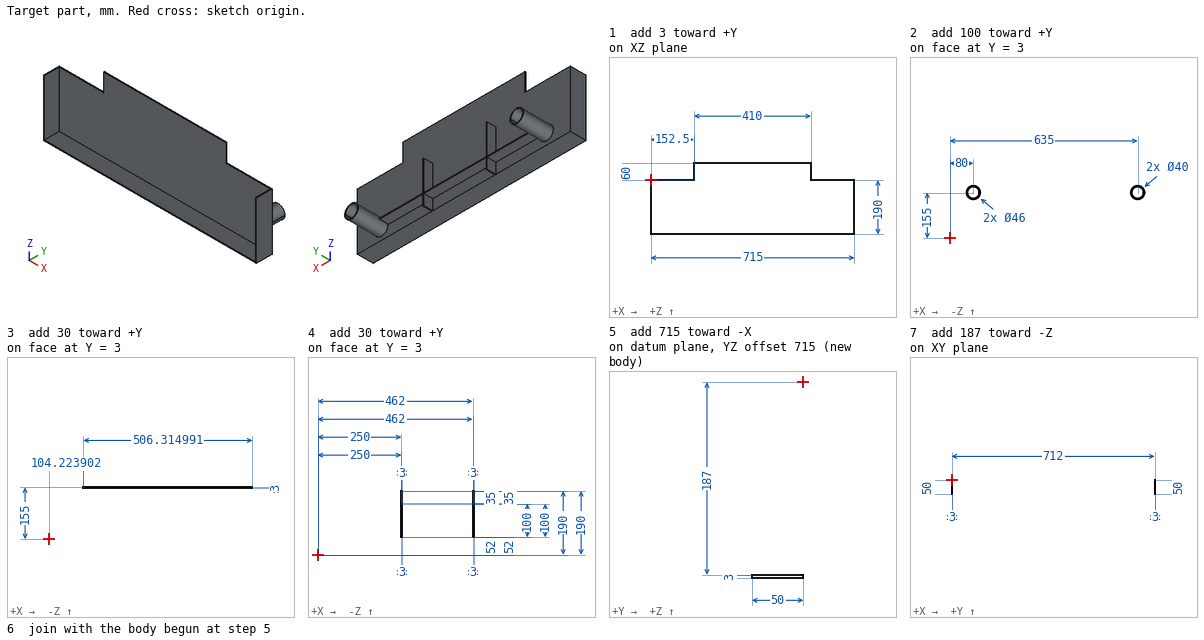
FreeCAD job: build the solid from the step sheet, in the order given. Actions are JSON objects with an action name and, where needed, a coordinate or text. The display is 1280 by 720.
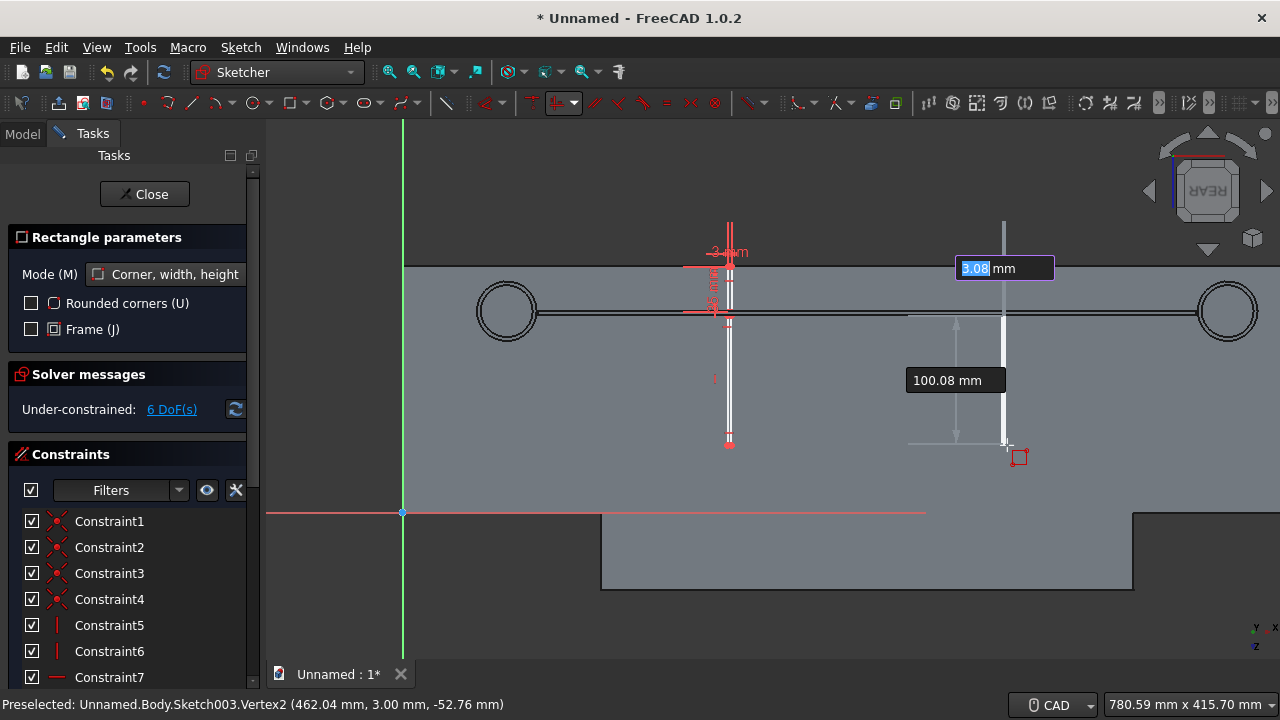
{"action": "type", "text": "3"}
{"action": "key", "text": "Tab"}
{"action": "type", "text": "100"}
{"action": "key", "text": "Return"}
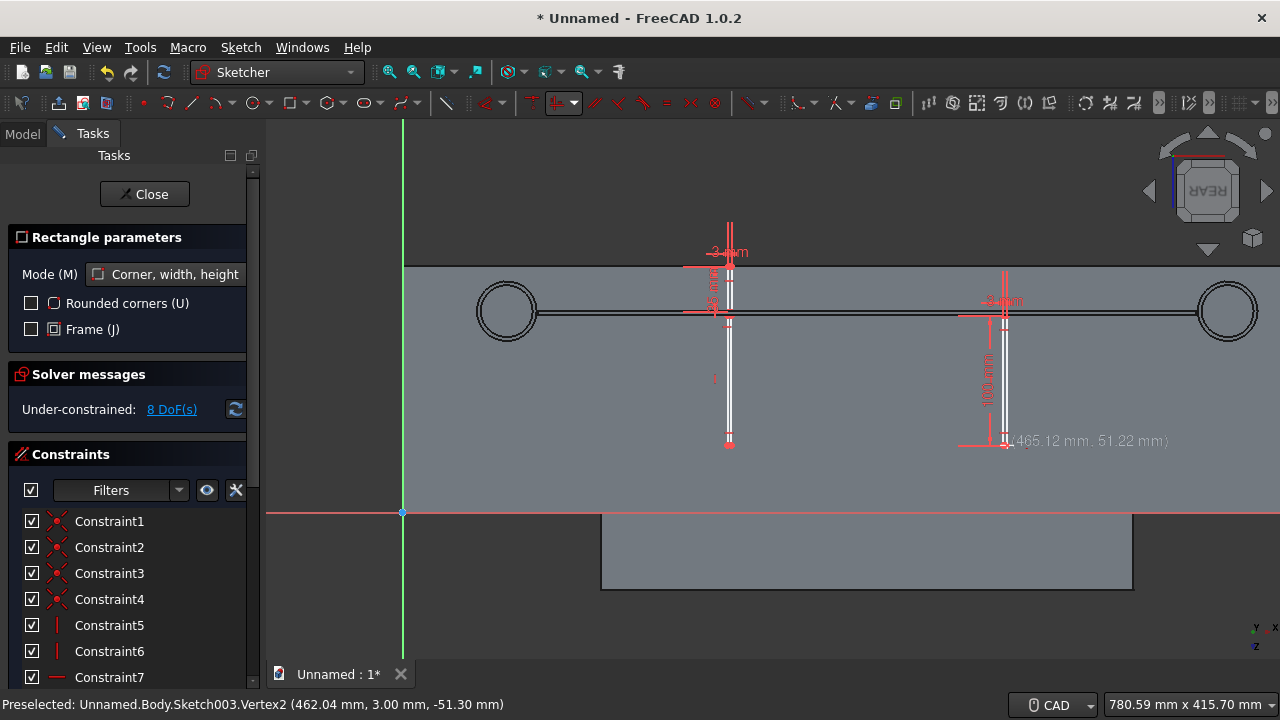
{"action": "scroll", "coordinate": [1003, 266], "scroll_direction": "up", "scroll_amount": 8}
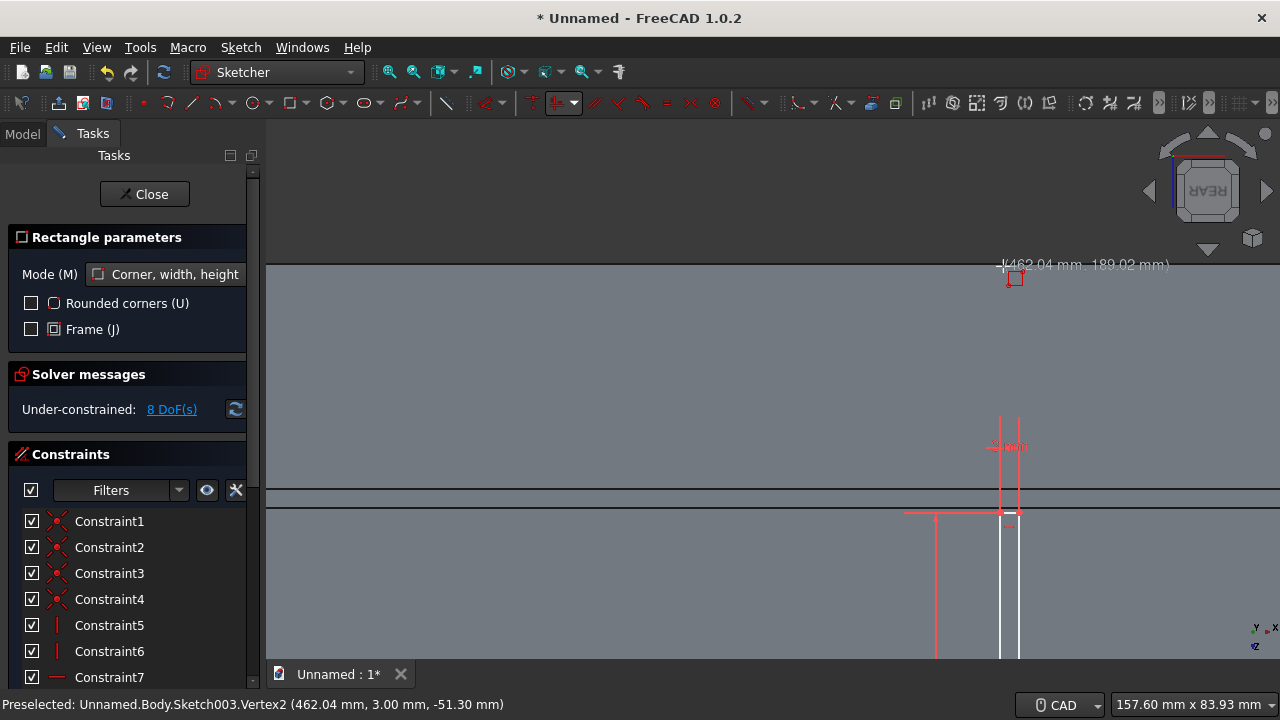
{"action": "scroll", "coordinate": [1003, 266], "scroll_direction": "down", "scroll_amount": 8}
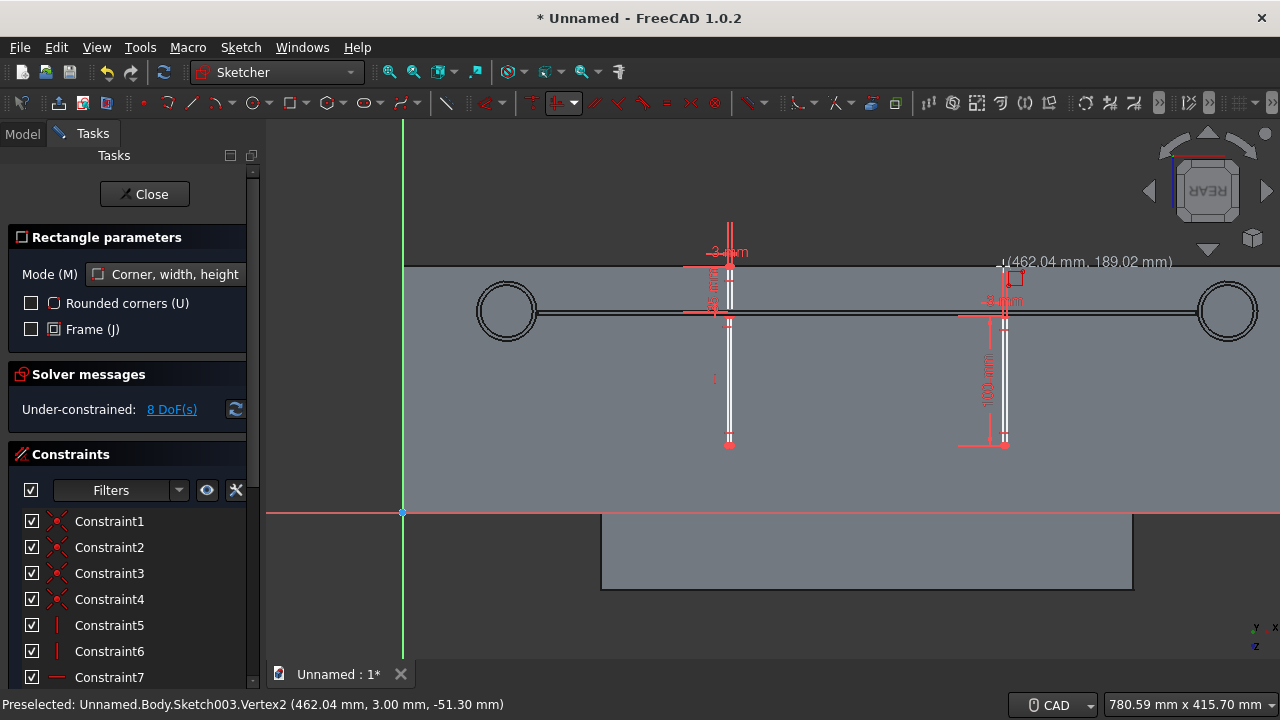
{"action": "left_click", "coordinate": [1003, 266]}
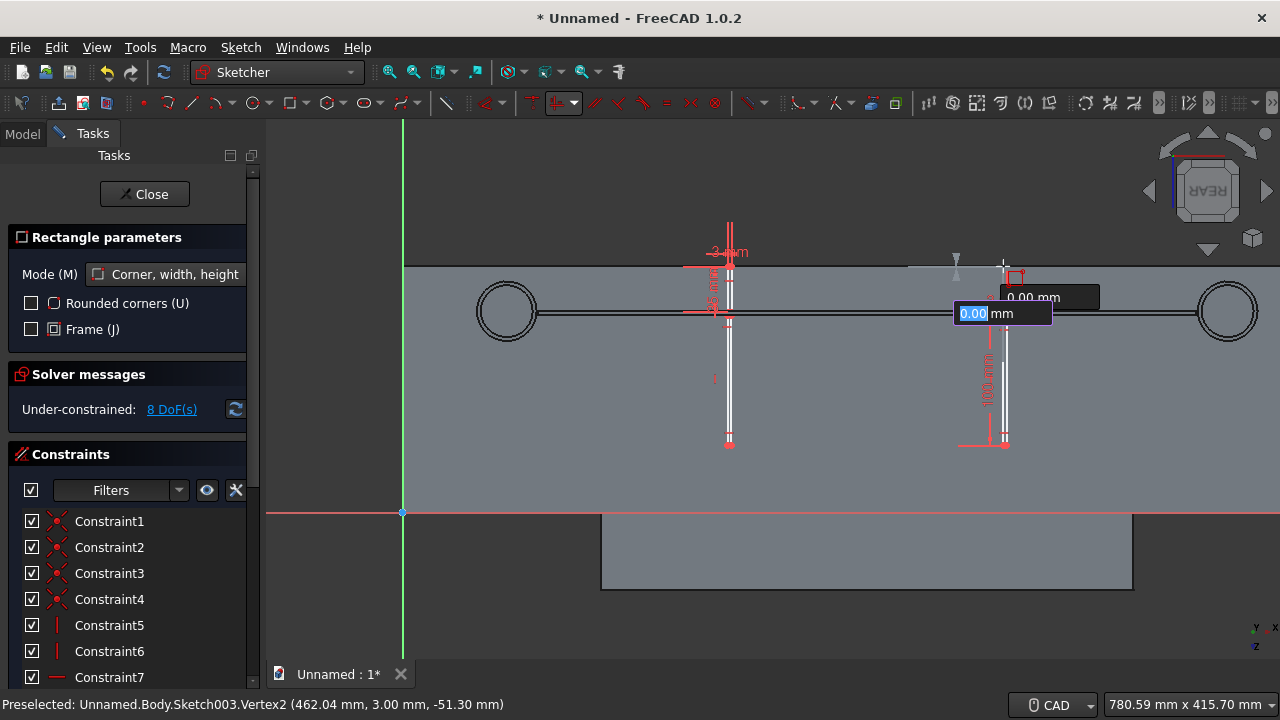
{"action": "scroll", "coordinate": [1007, 311], "scroll_direction": "up", "scroll_amount": 8}
{"action": "mouse_move", "coordinate": [1003, 311]}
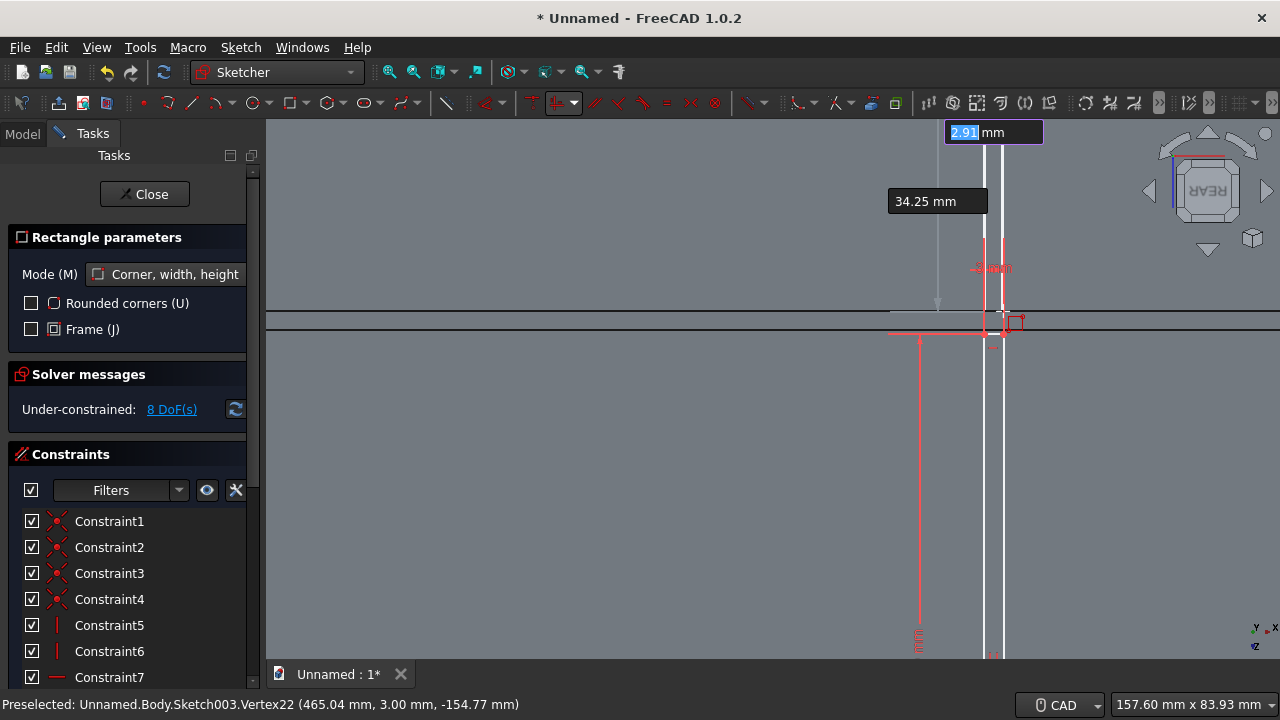
{"action": "type", "text": "3"}
{"action": "key", "text": "Tab"}
{"action": "type", "text": "35"}
{"action": "key", "text": "Return"}
{"action": "key", "text": "Escape"}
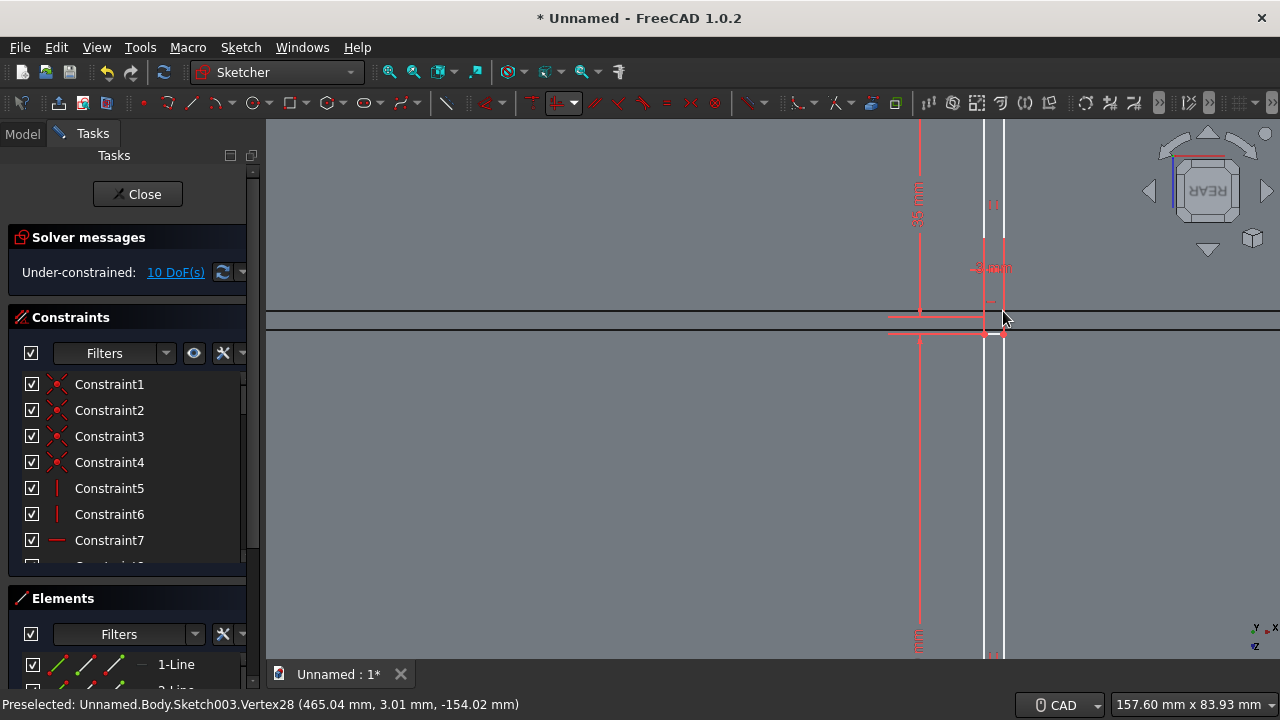
{"action": "left_click", "coordinate": [486, 104]}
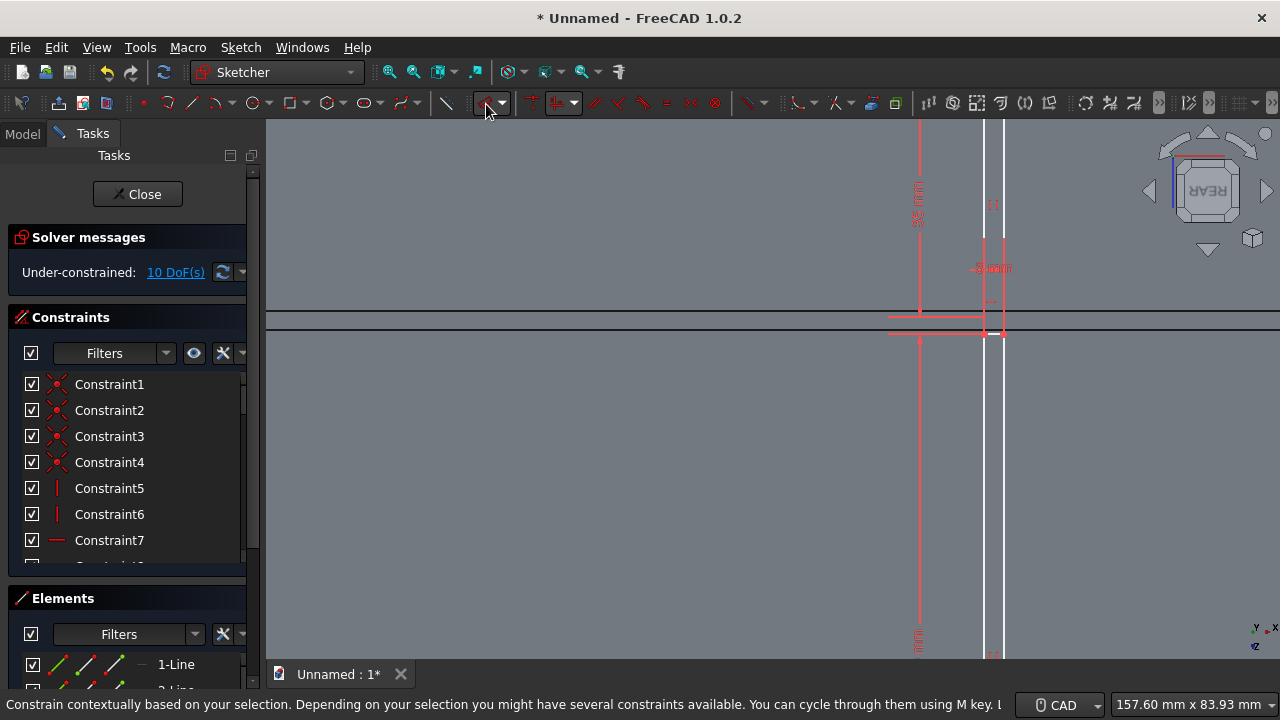
{"action": "scroll", "coordinate": [1007, 311], "scroll_direction": "down", "scroll_amount": 8}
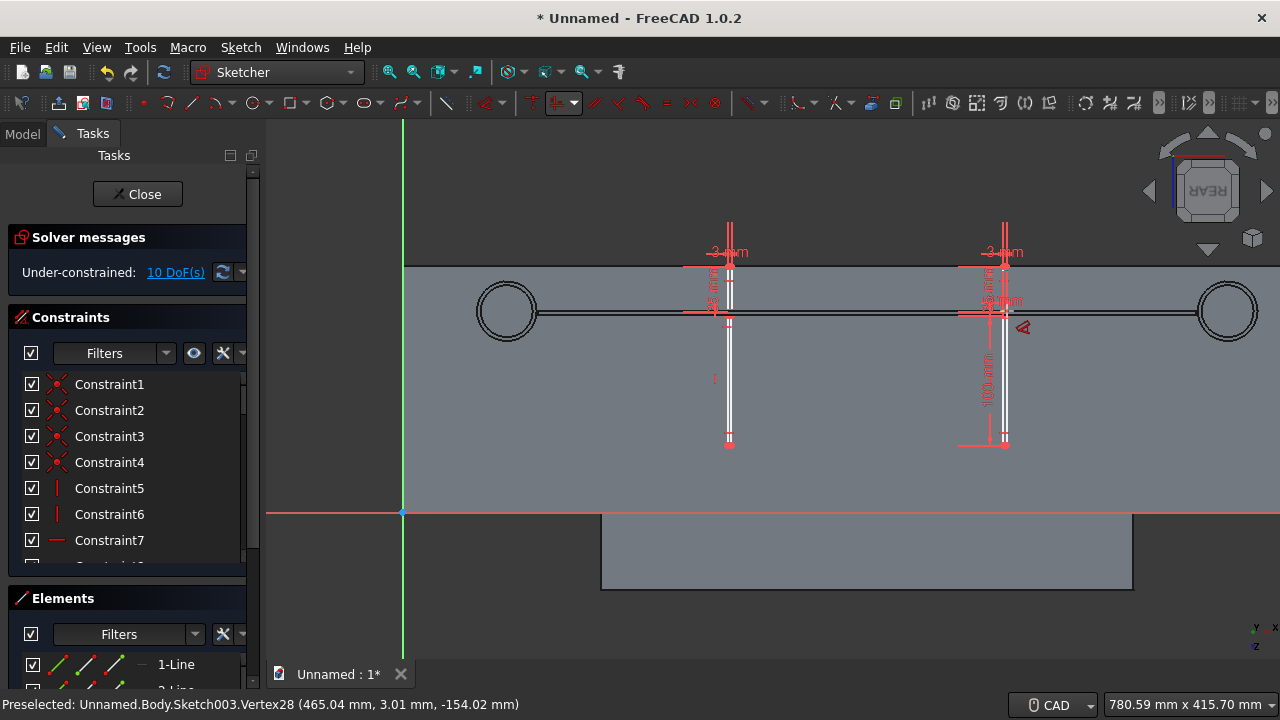
{"action": "scroll", "coordinate": [729, 446], "scroll_direction": "up", "scroll_amount": 12}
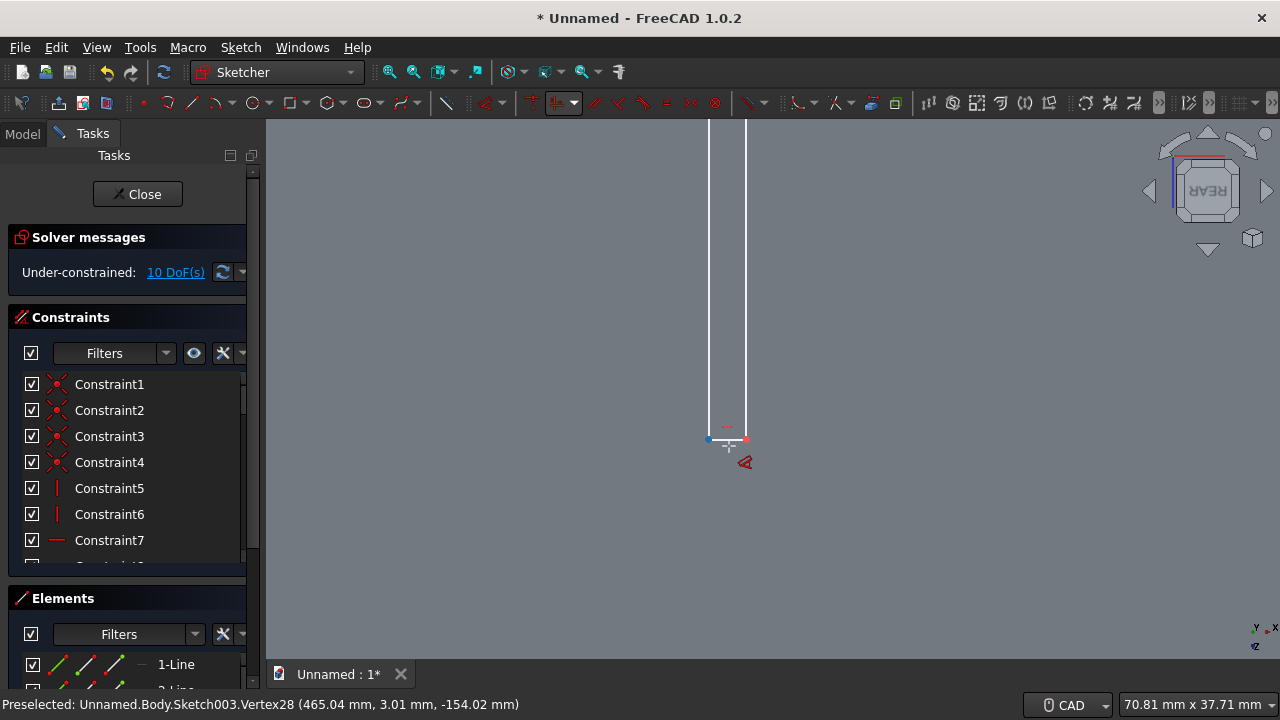
{"action": "left_click", "coordinate": [727, 440]}
{"action": "left_click", "coordinate": [727, 474]}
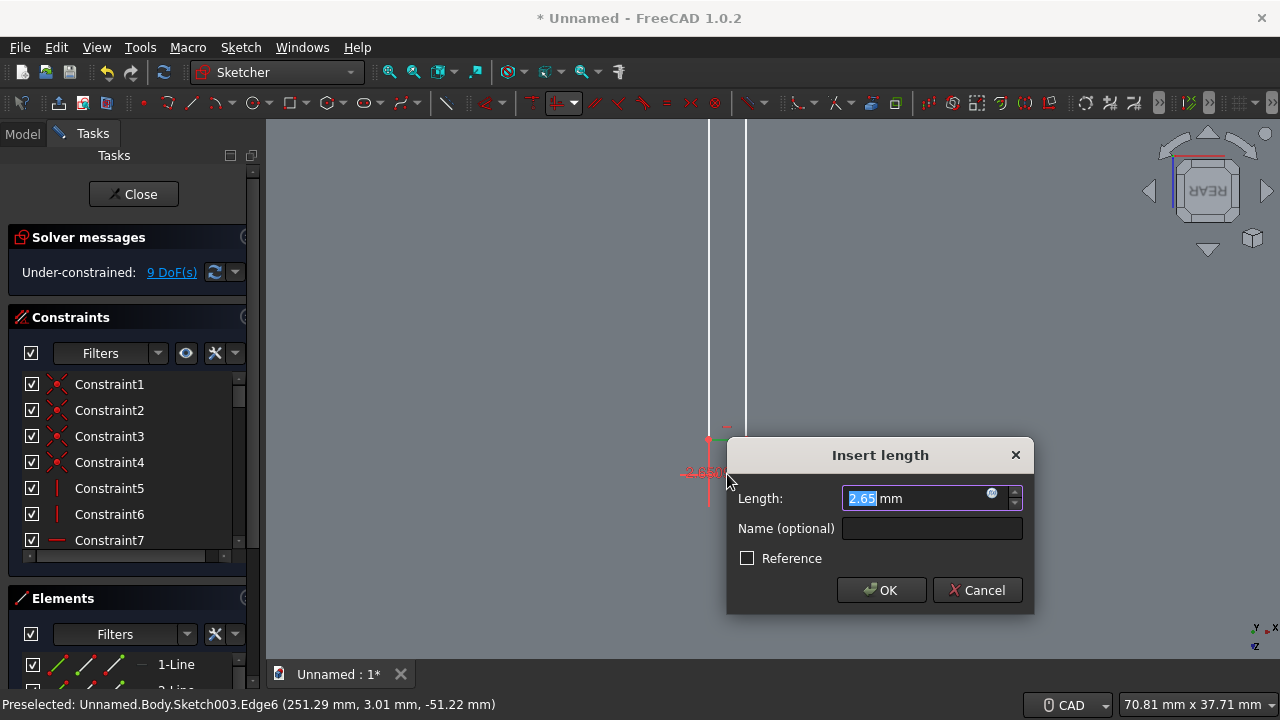
{"action": "type", "text": "3"}
{"action": "key", "text": "Return"}